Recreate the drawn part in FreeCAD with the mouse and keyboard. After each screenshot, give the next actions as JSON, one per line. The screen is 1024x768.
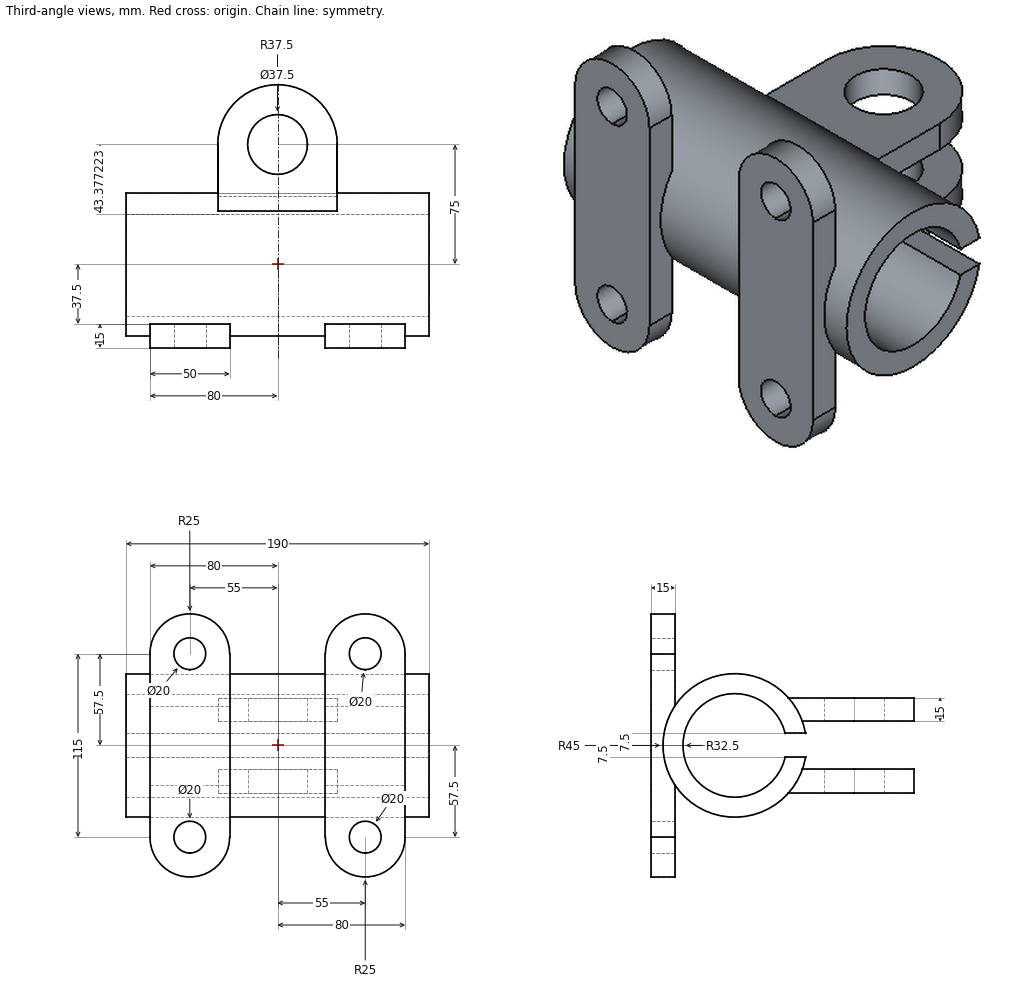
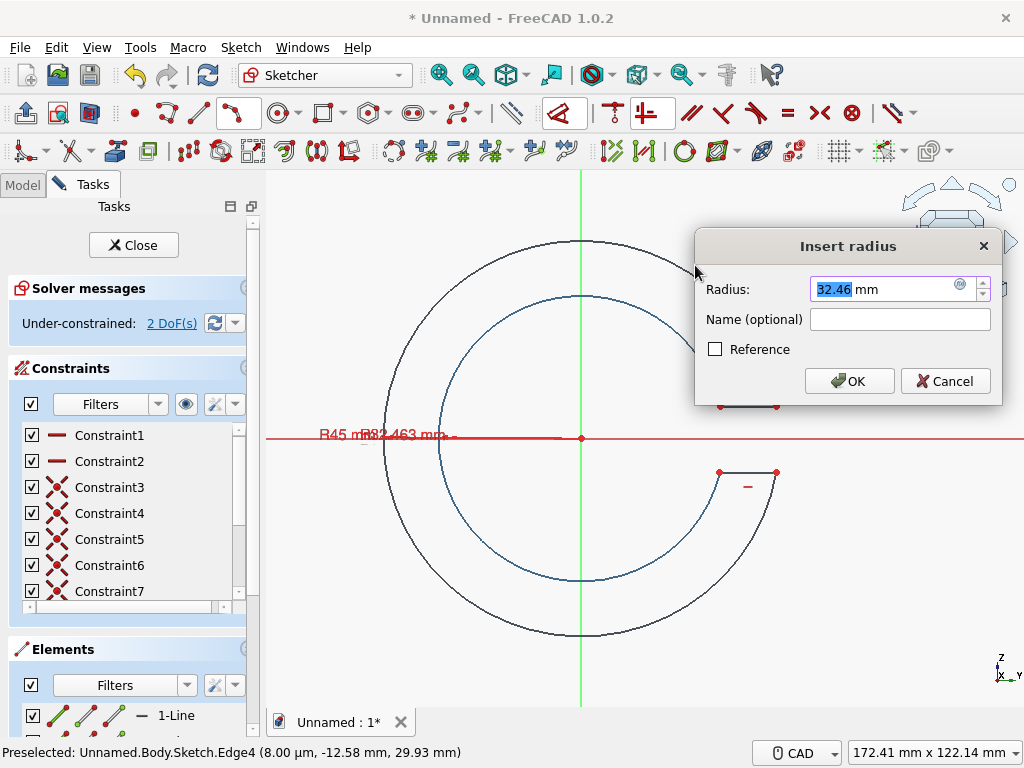
{"action": "type", "text": "32.5"}
{"action": "key", "text": "Return"}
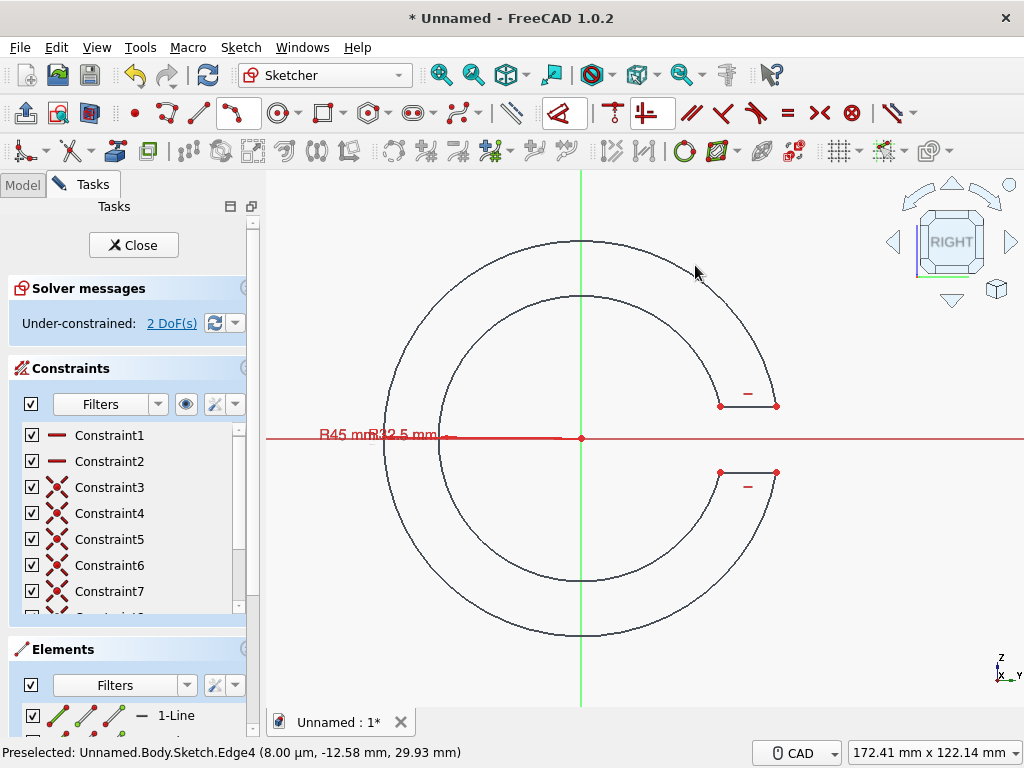
{"action": "left_click", "coordinate": [721, 407]}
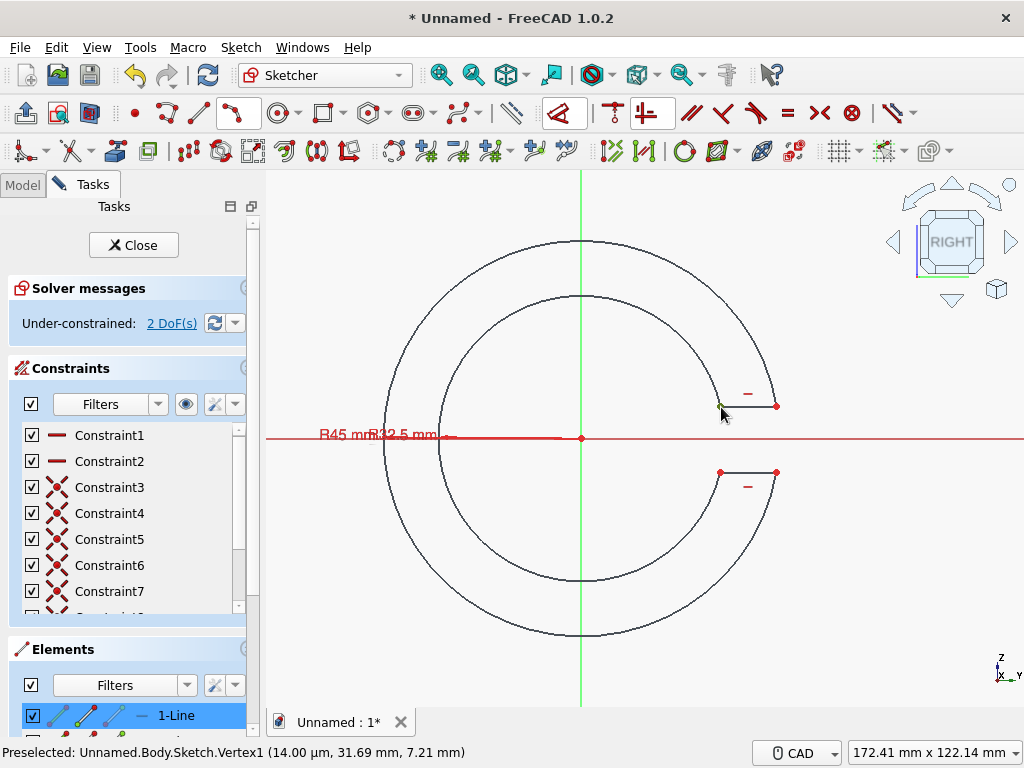
{"action": "left_click", "coordinate": [582, 114]}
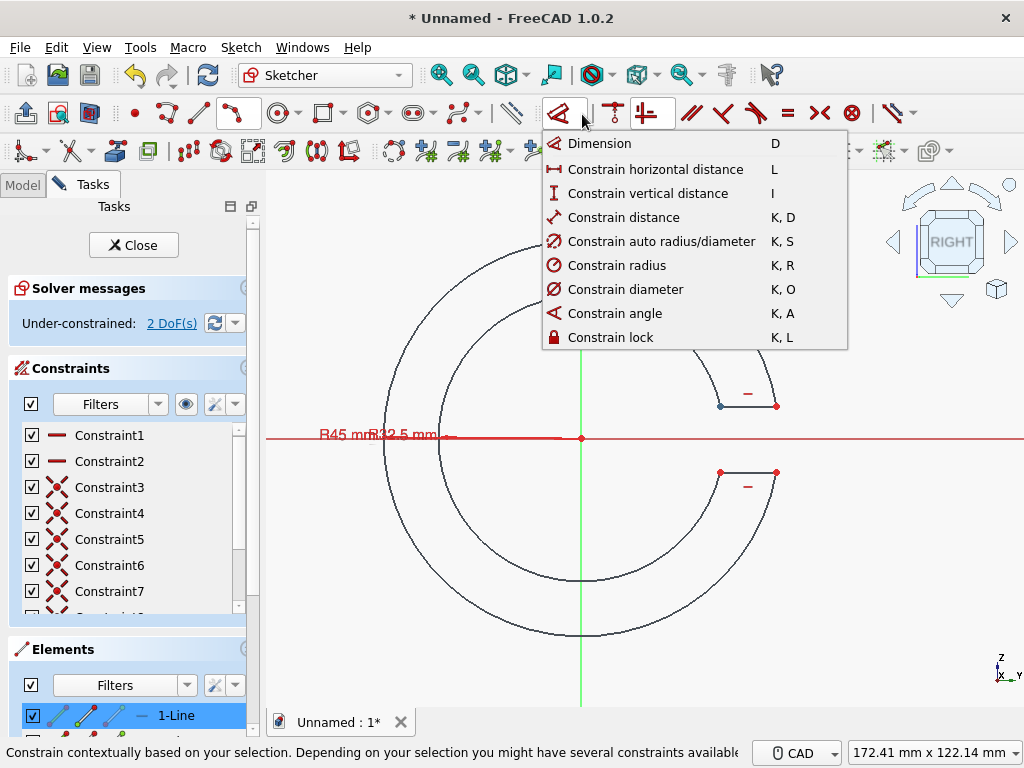
{"action": "left_click", "coordinate": [695, 193]}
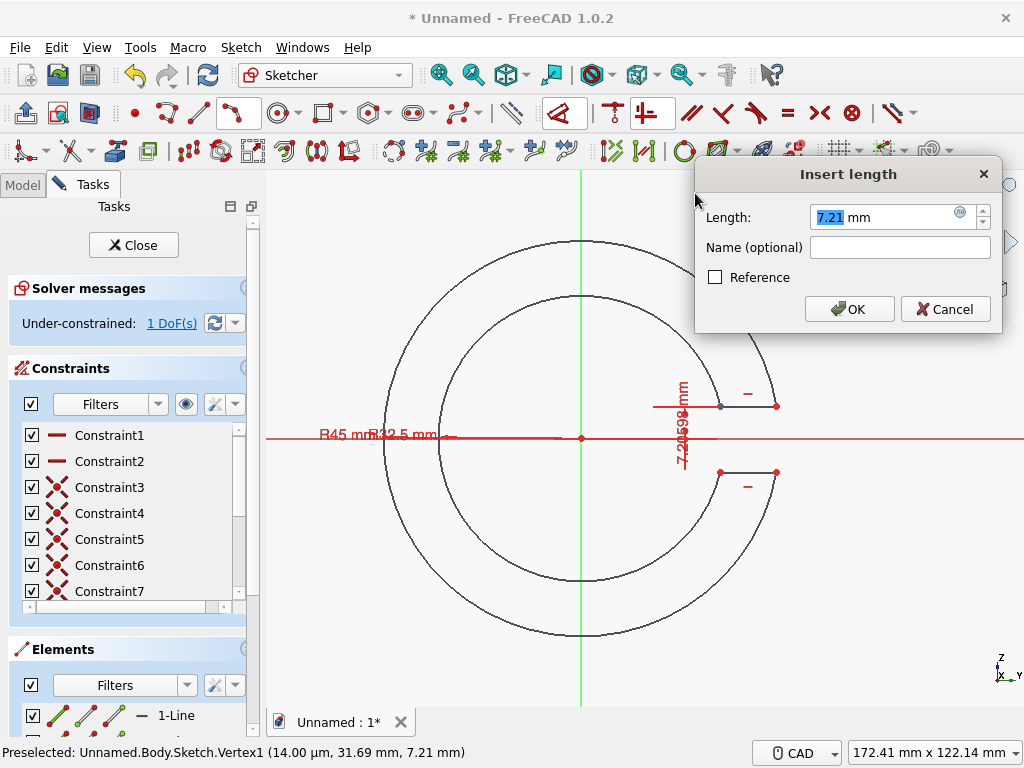
{"action": "type", "text": "7.5"}
{"action": "key", "text": "Return"}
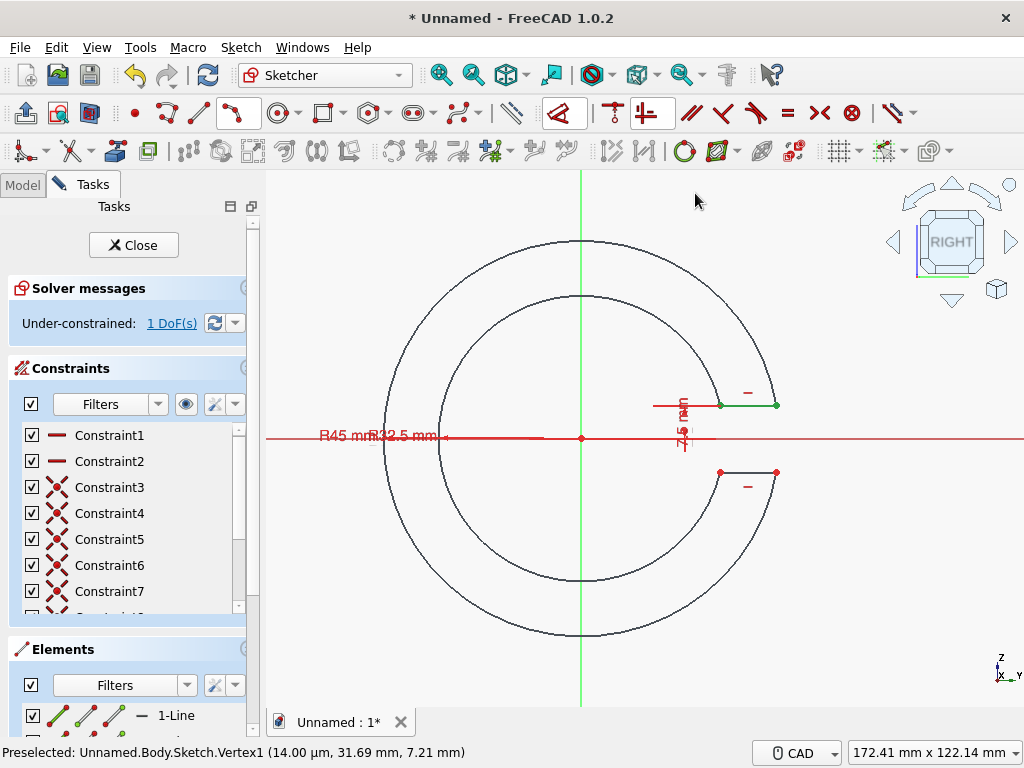
{"action": "left_click", "coordinate": [776, 473]}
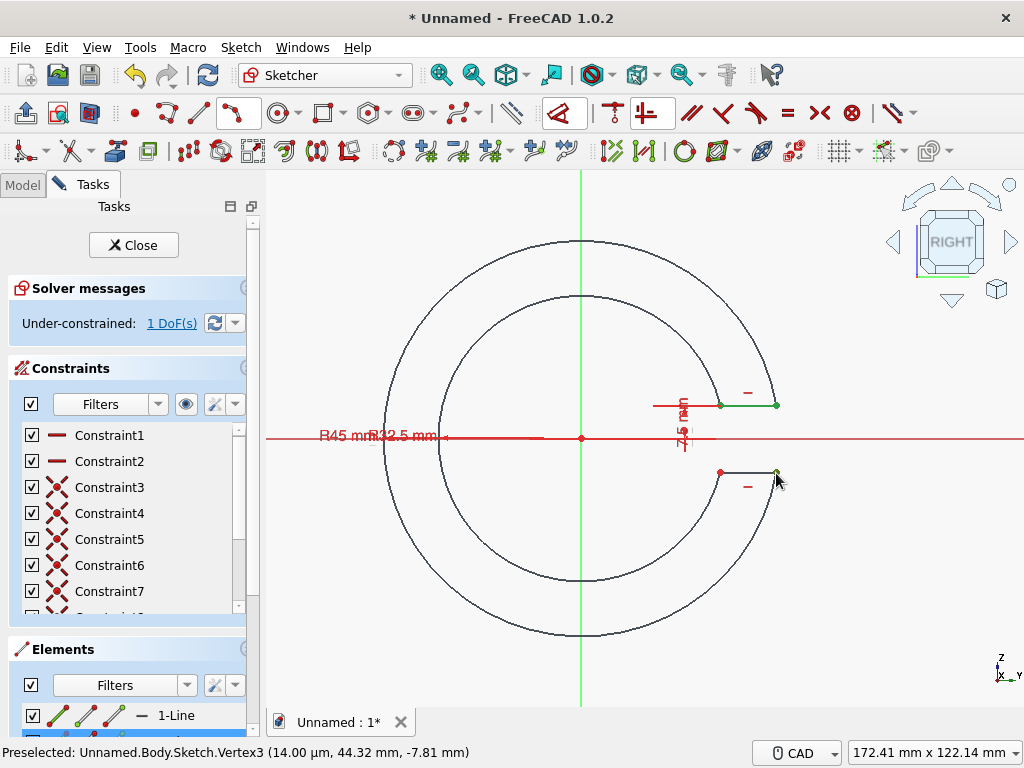
{"action": "left_click", "coordinate": [582, 114]}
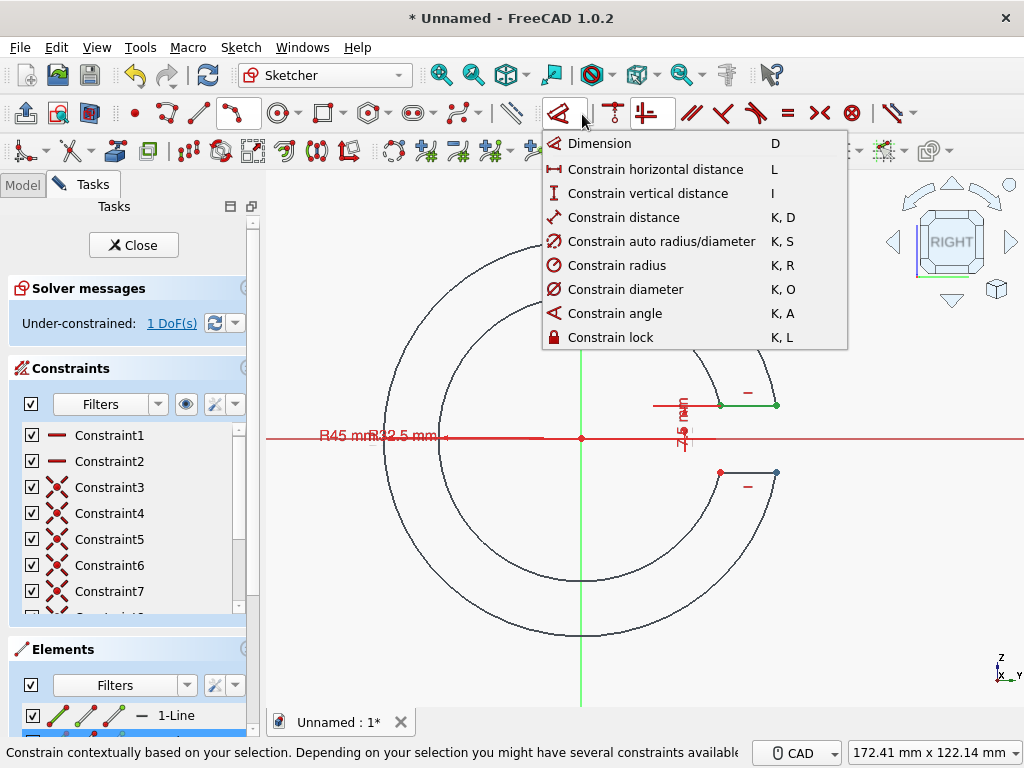
{"action": "left_click", "coordinate": [695, 193]}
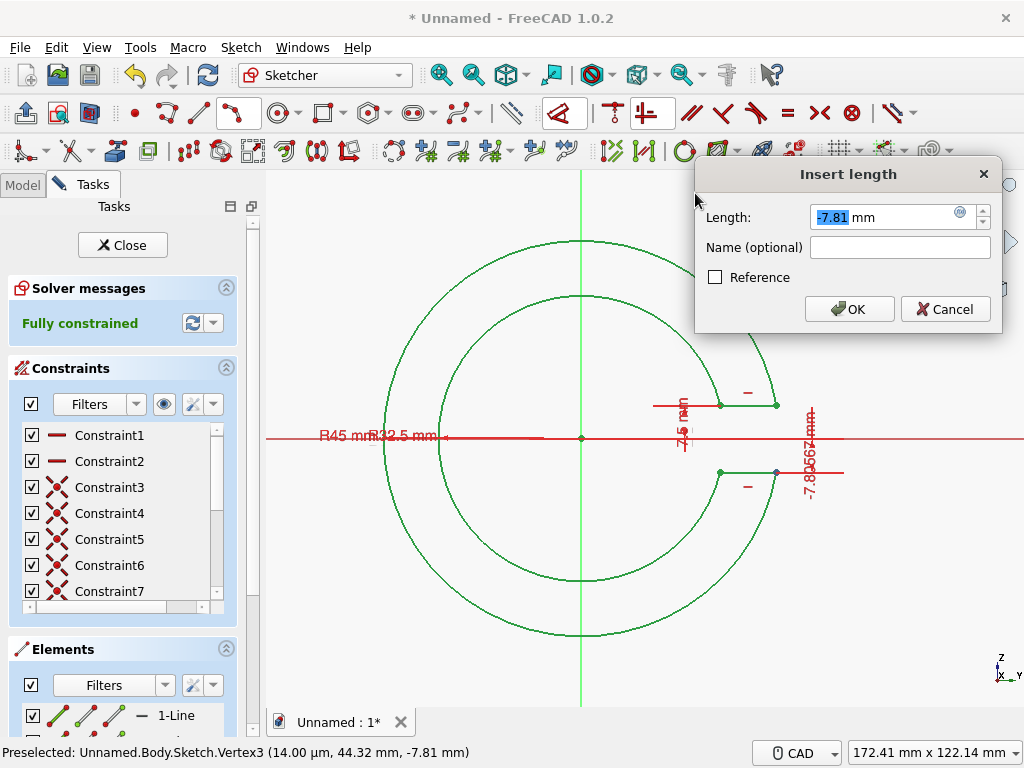
{"action": "type", "text": "-7.5"}
{"action": "key", "text": "Return"}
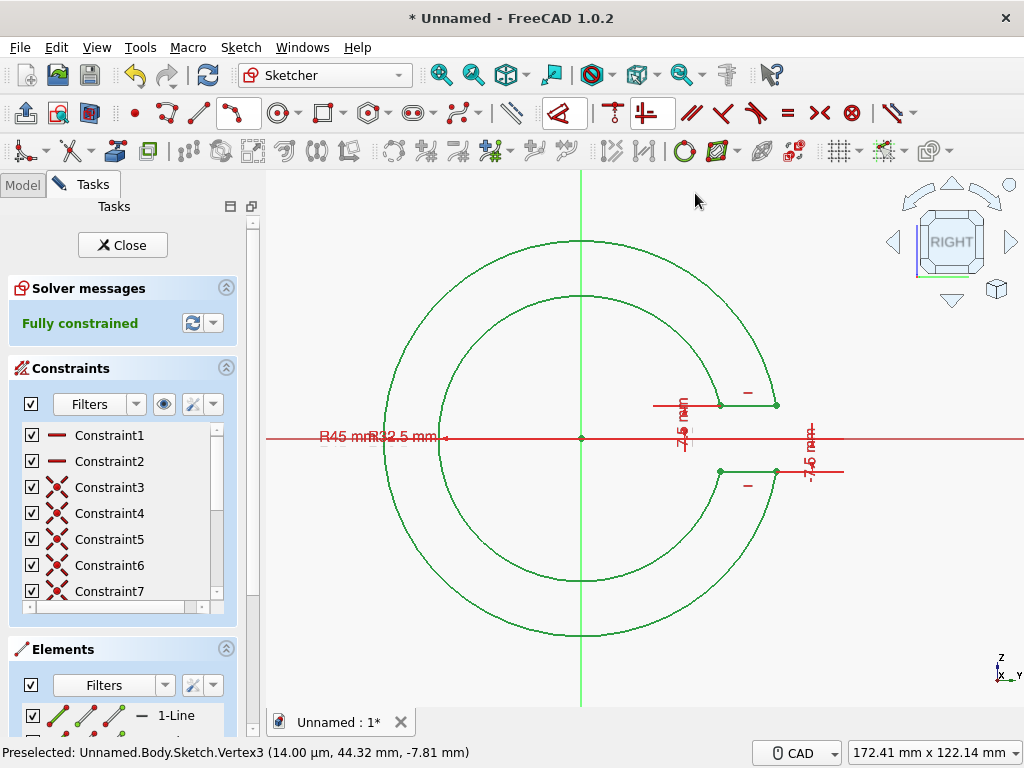
{"action": "left_click", "coordinate": [123, 245]}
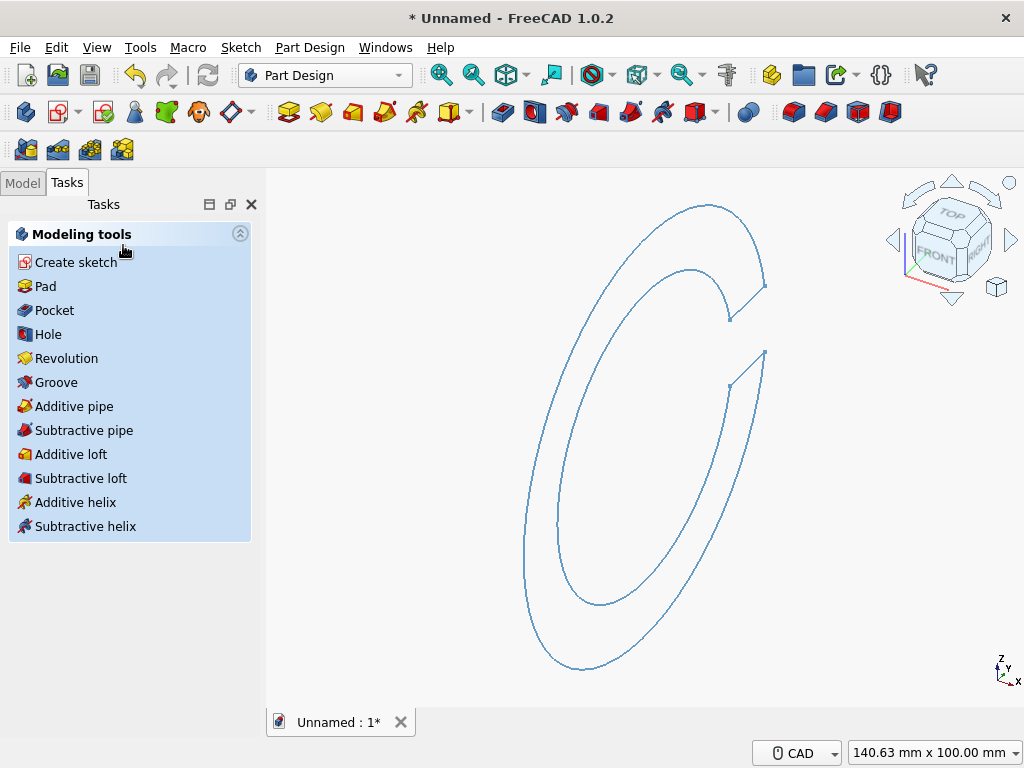
{"action": "left_click", "coordinate": [290, 112]}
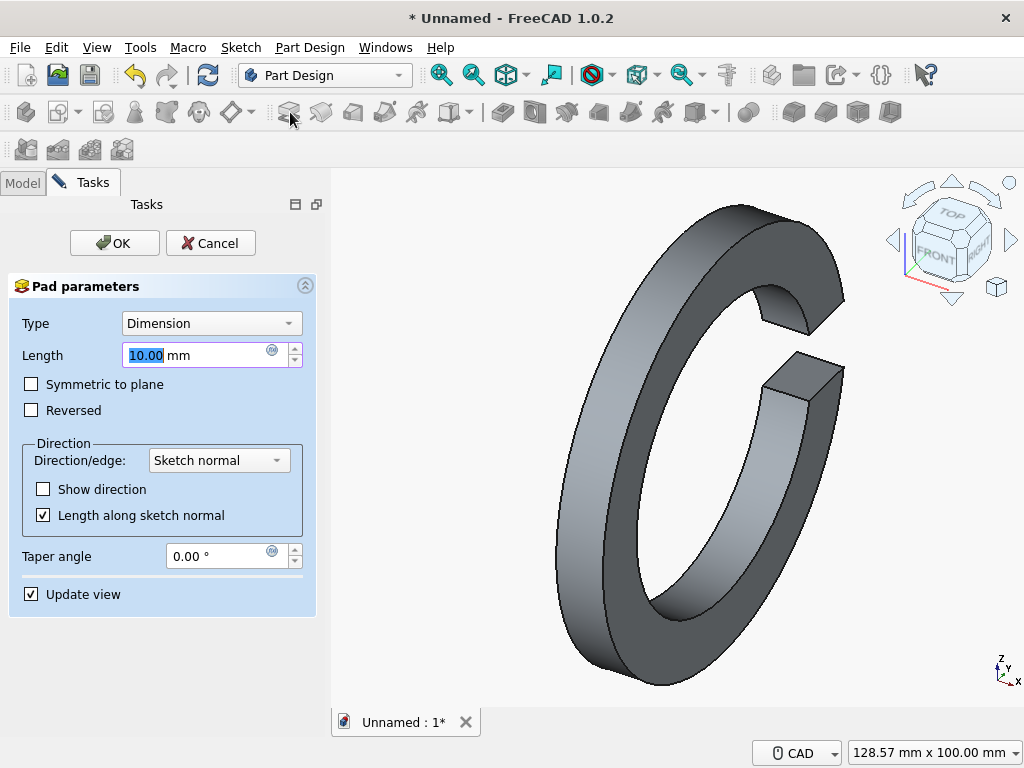
{"action": "type", "text": "190"}
{"action": "key", "text": "Tab"}